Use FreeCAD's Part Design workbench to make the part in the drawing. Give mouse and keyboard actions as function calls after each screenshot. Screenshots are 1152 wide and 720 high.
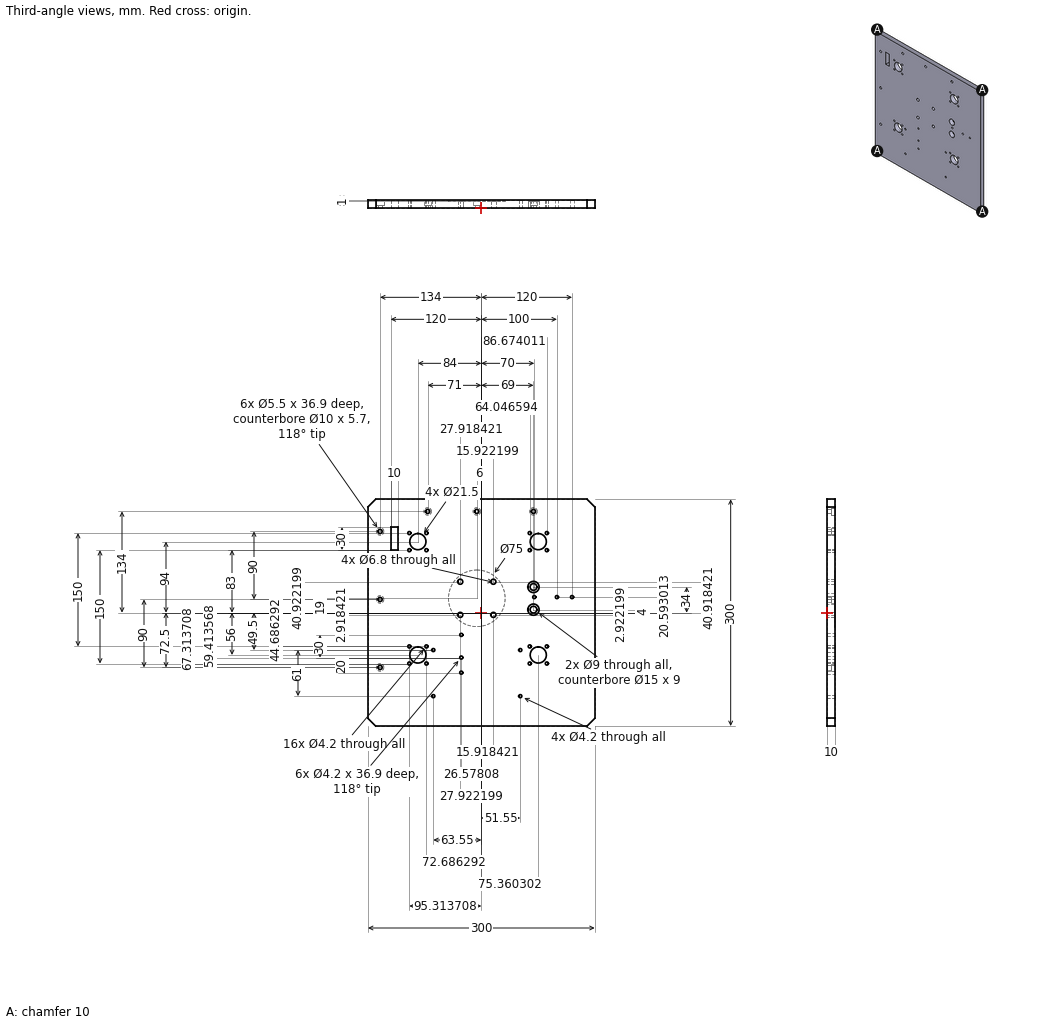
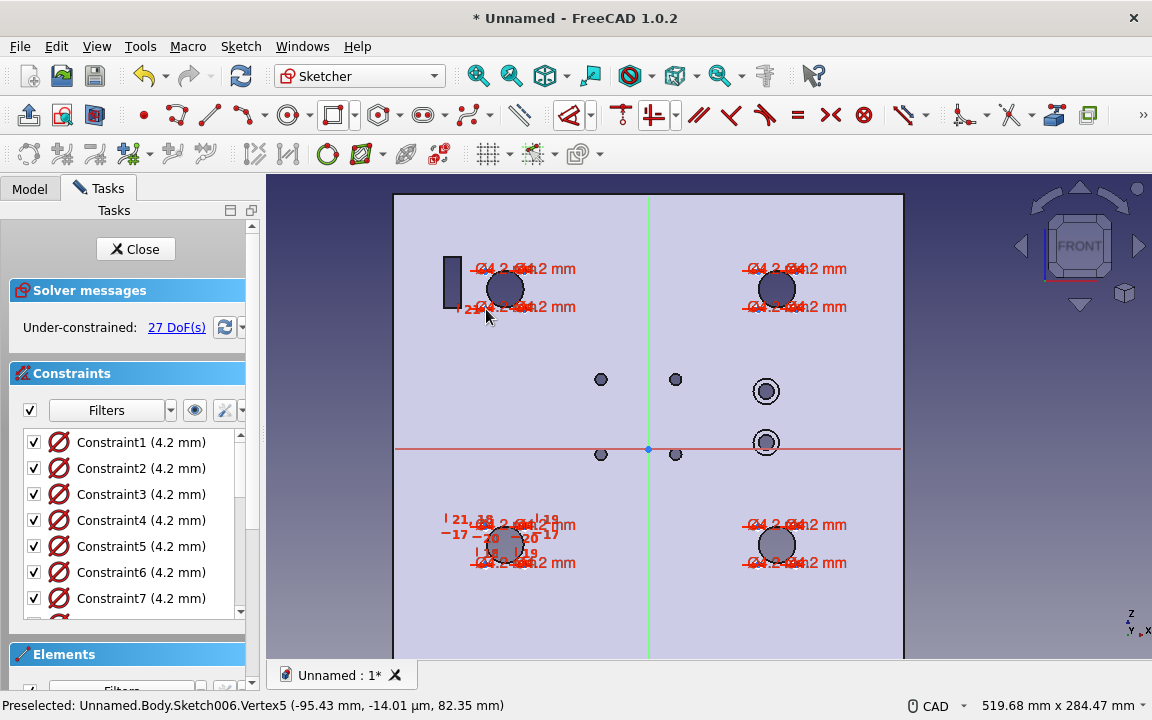
click(486, 309)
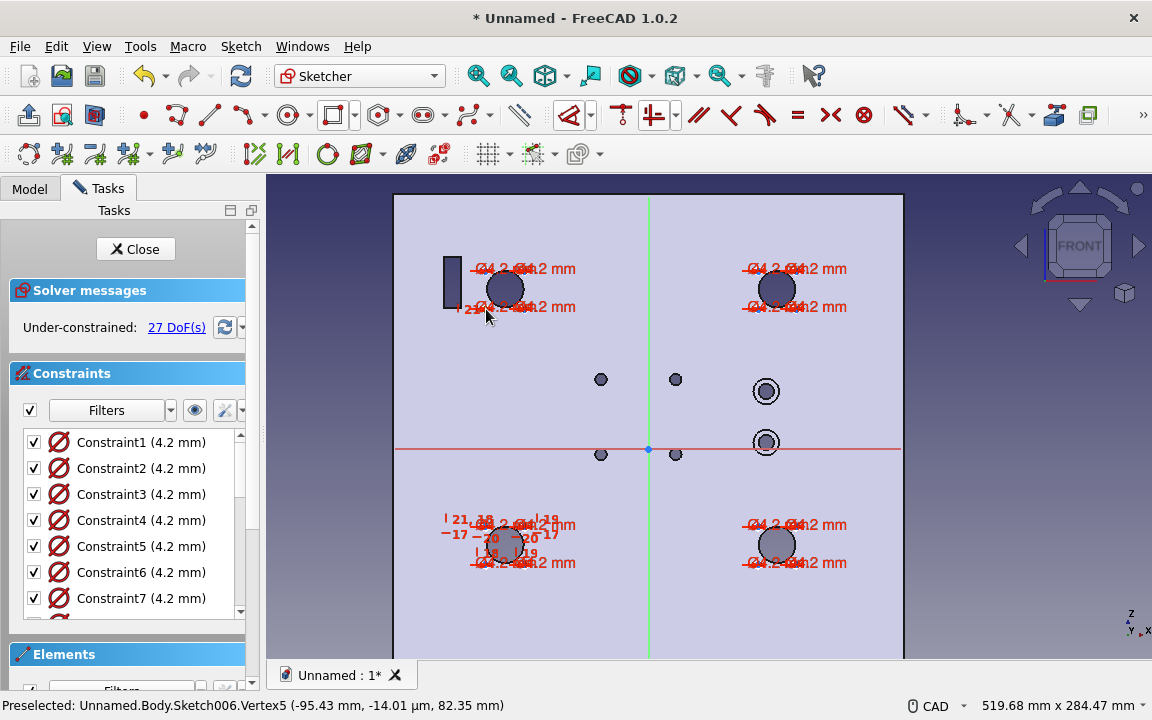
click(486, 271)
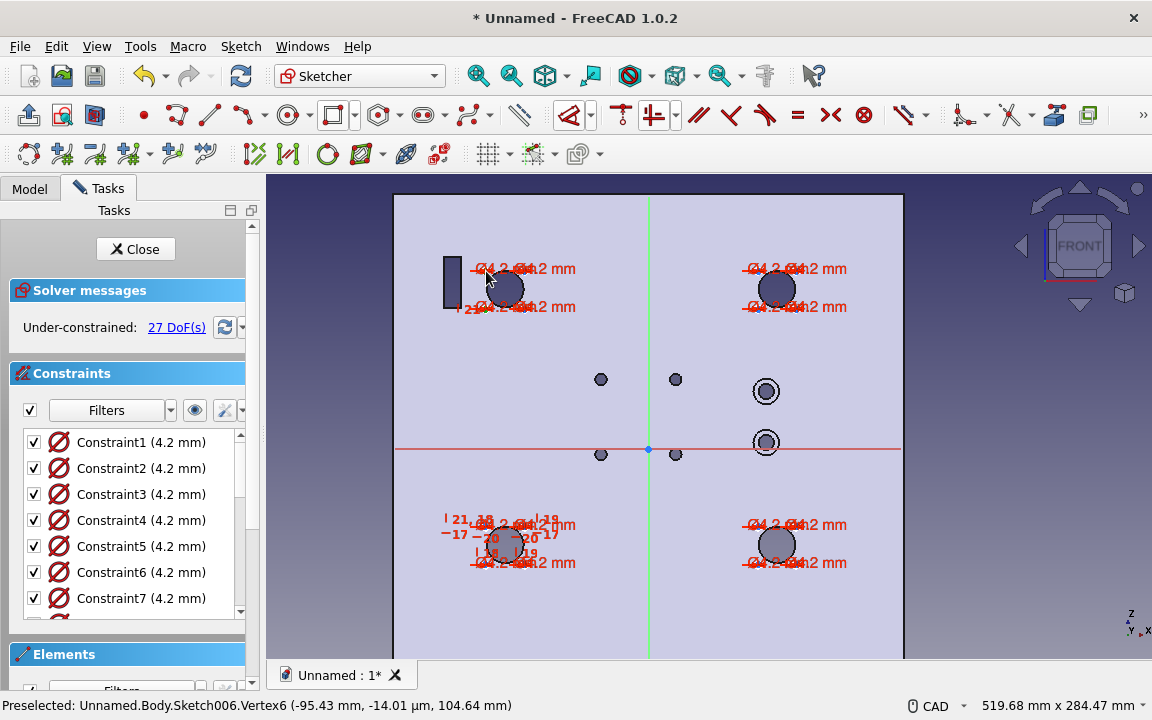
click(676, 116)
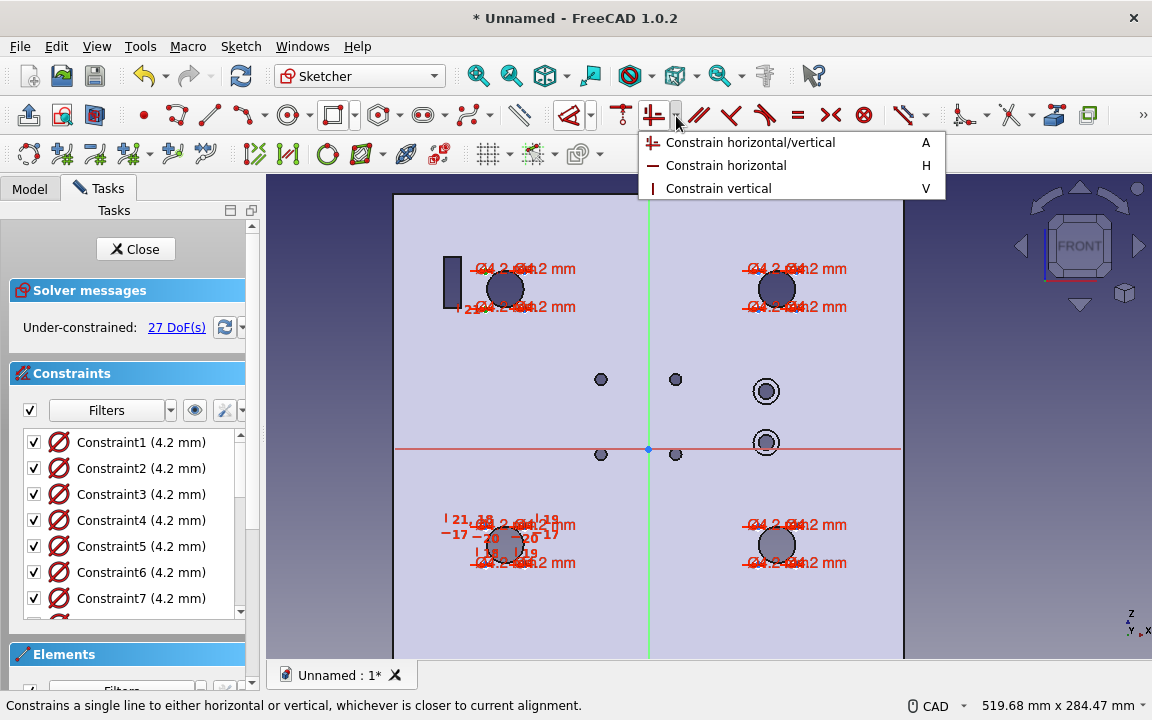
click(792, 188)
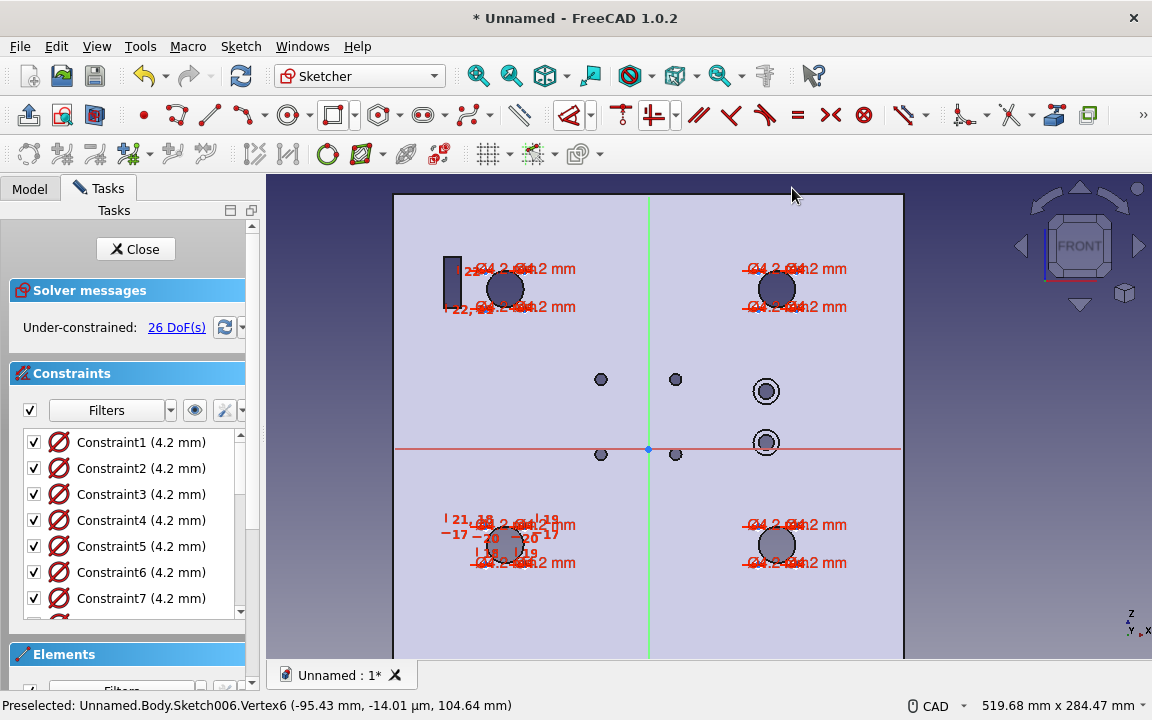
click(525, 527)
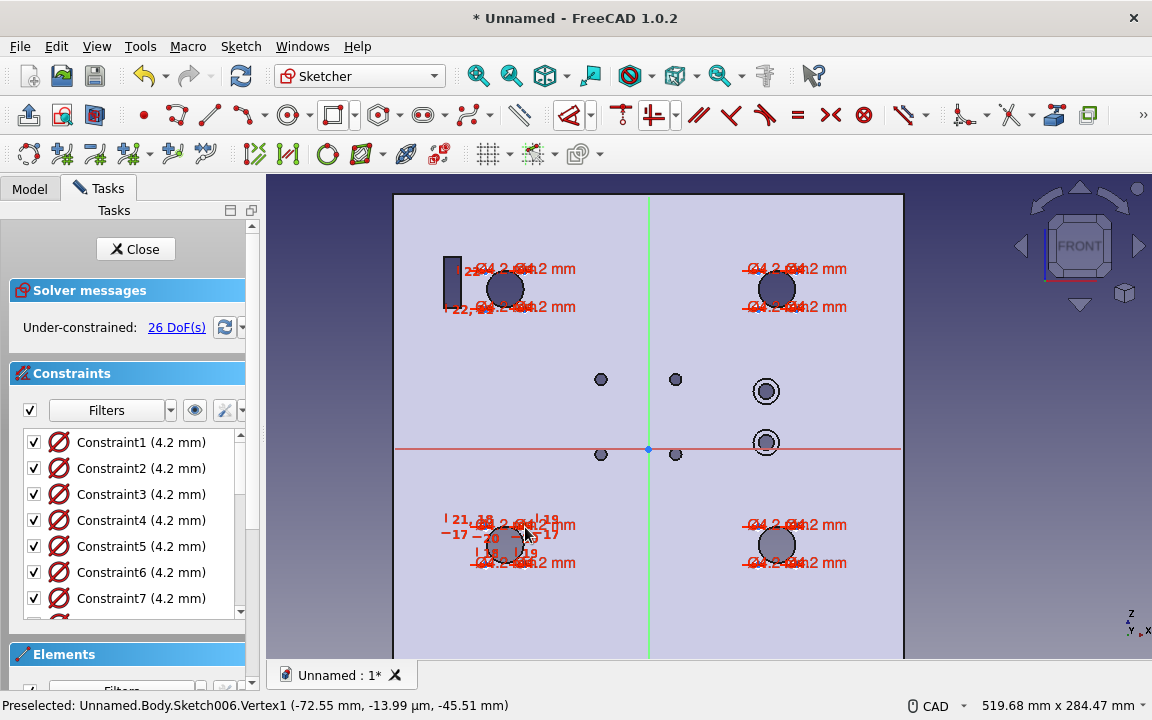
click(525, 271)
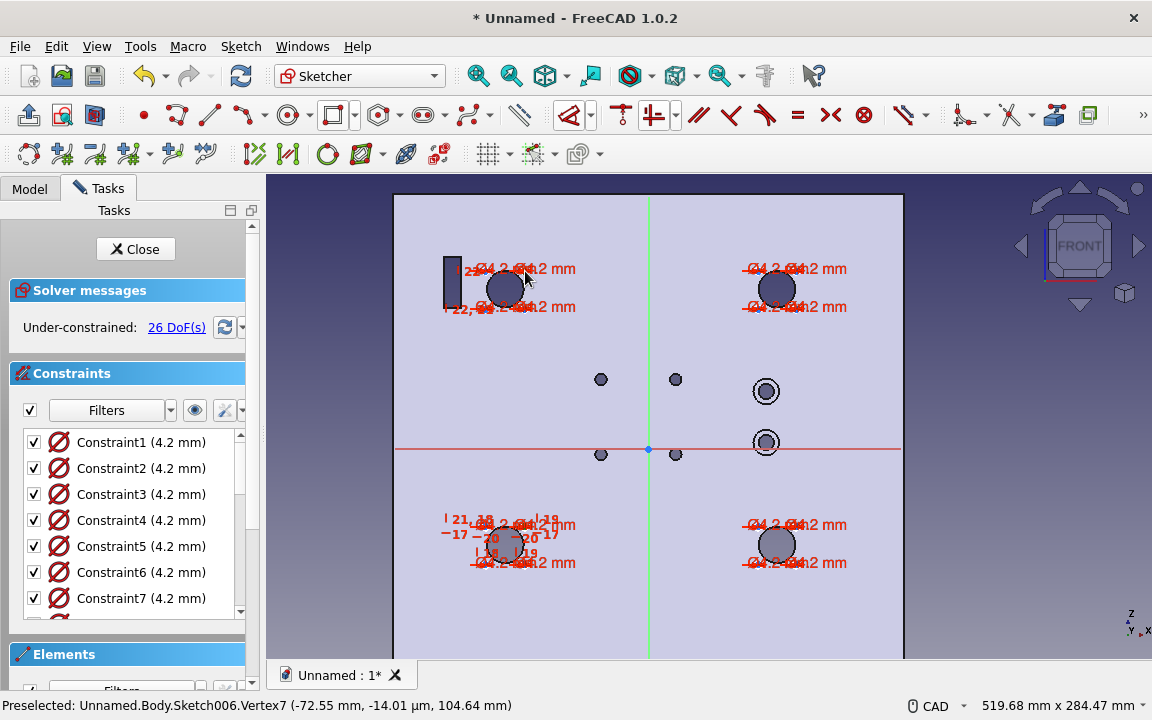
key(v)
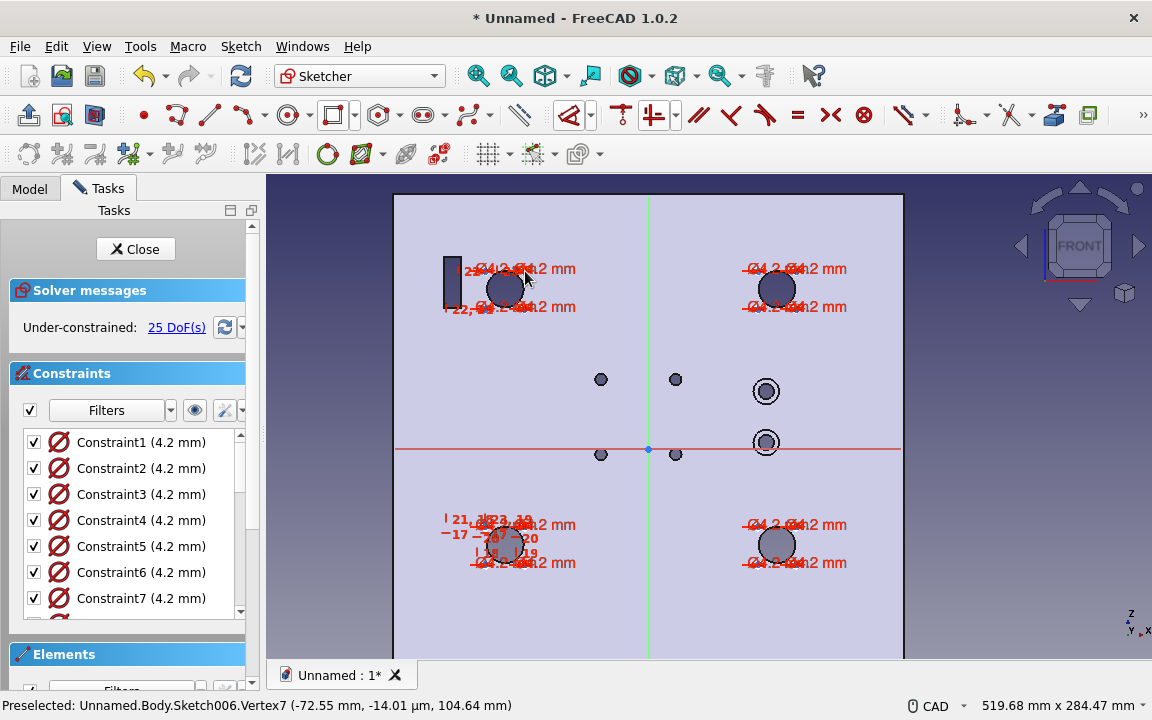
click(486, 271)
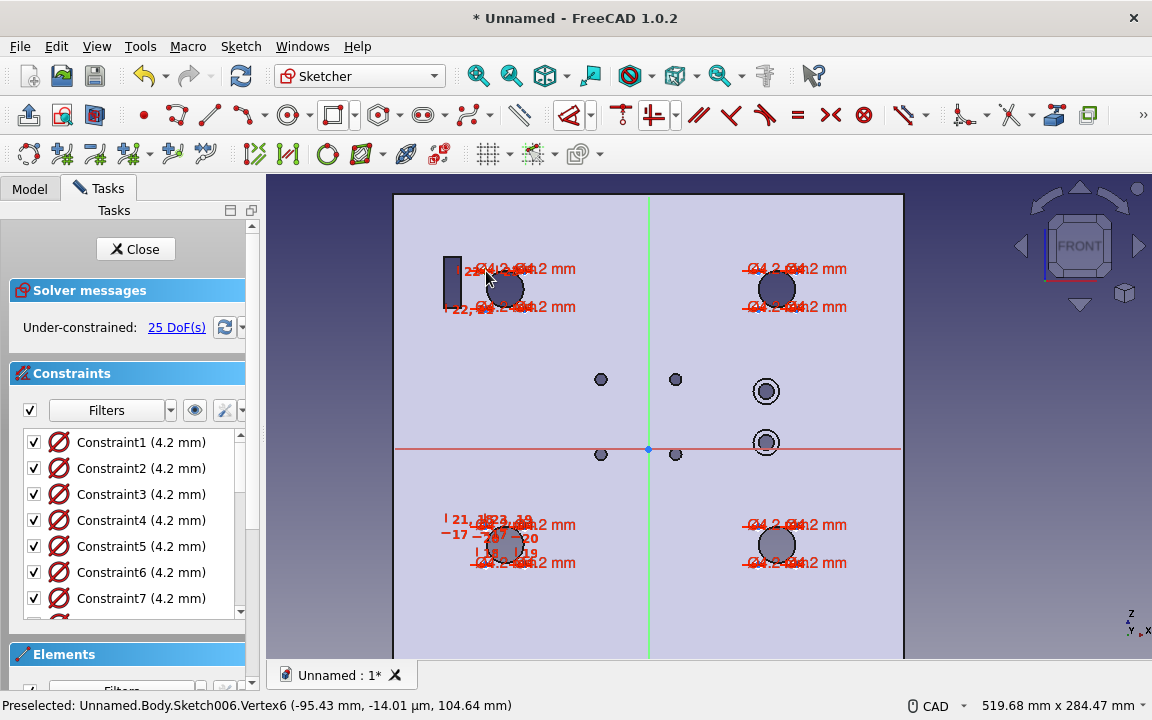
click(525, 271)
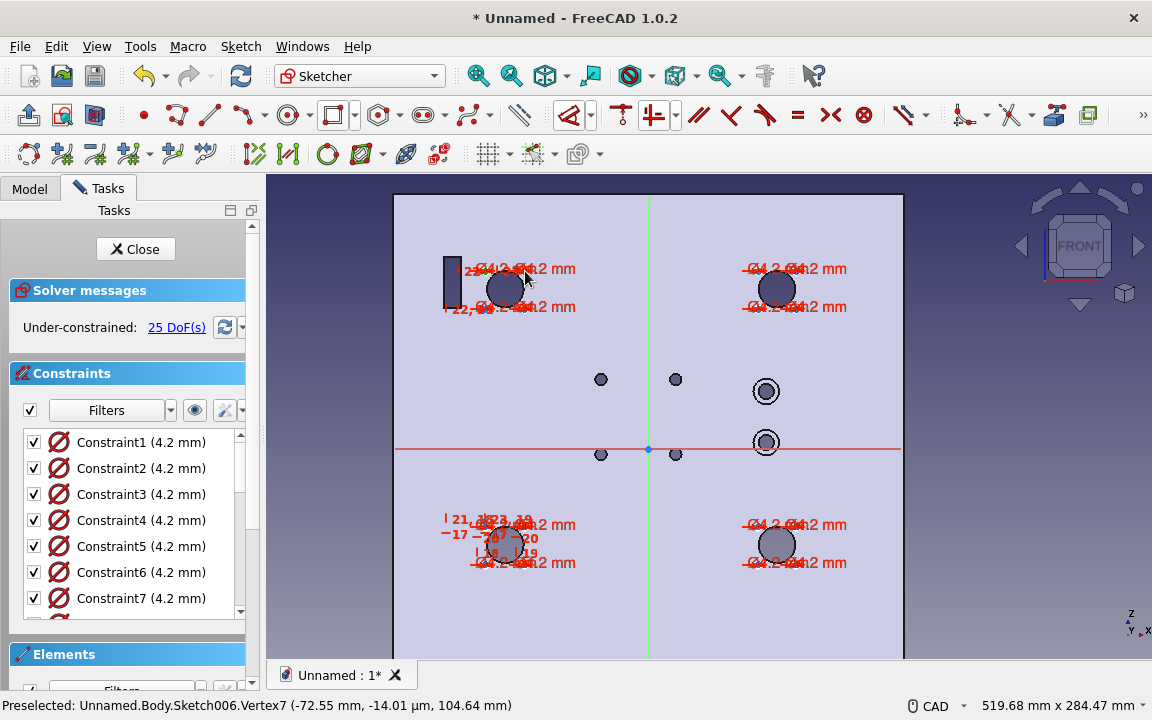
click(676, 116)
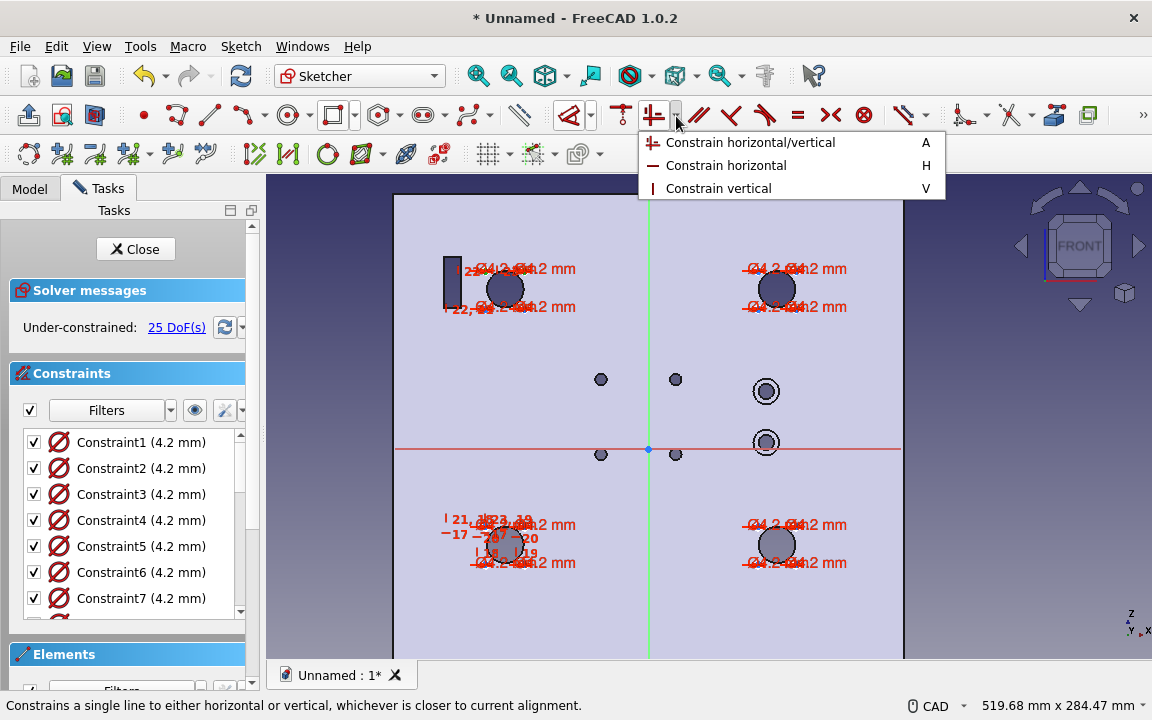
click(792, 166)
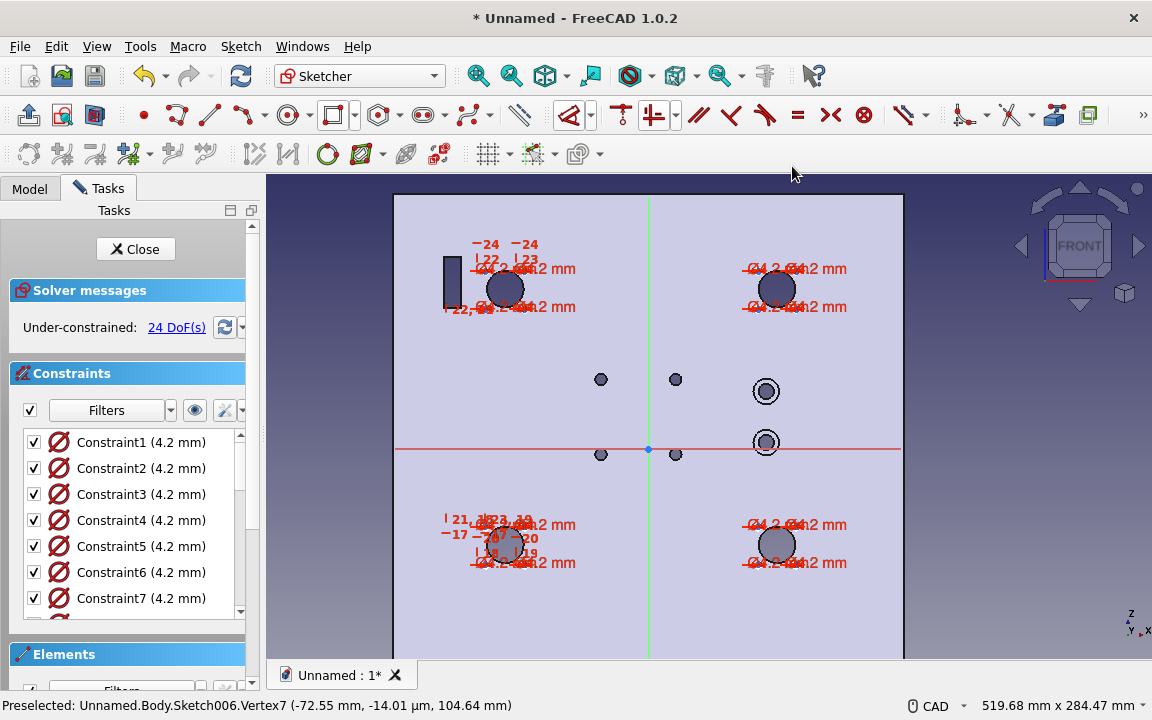
click(525, 271)